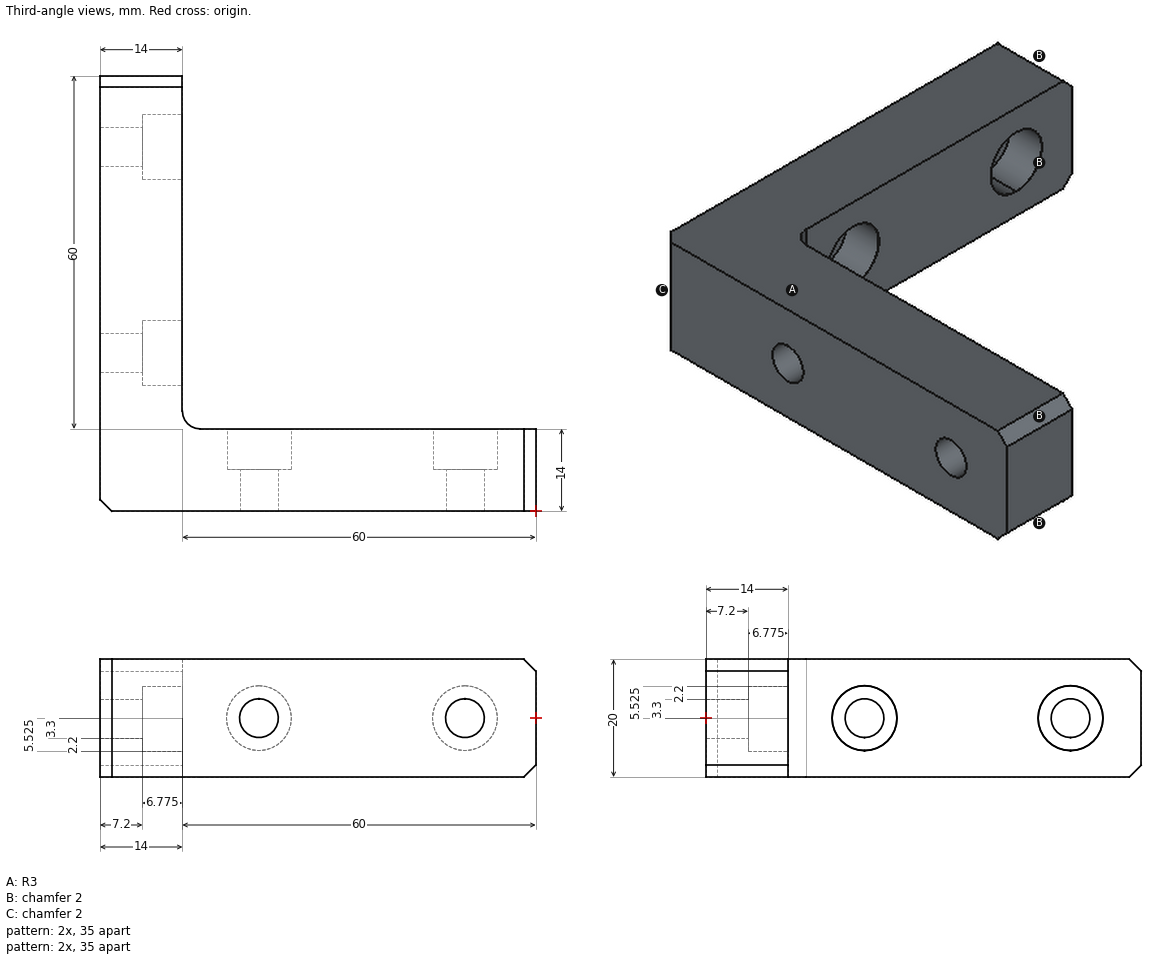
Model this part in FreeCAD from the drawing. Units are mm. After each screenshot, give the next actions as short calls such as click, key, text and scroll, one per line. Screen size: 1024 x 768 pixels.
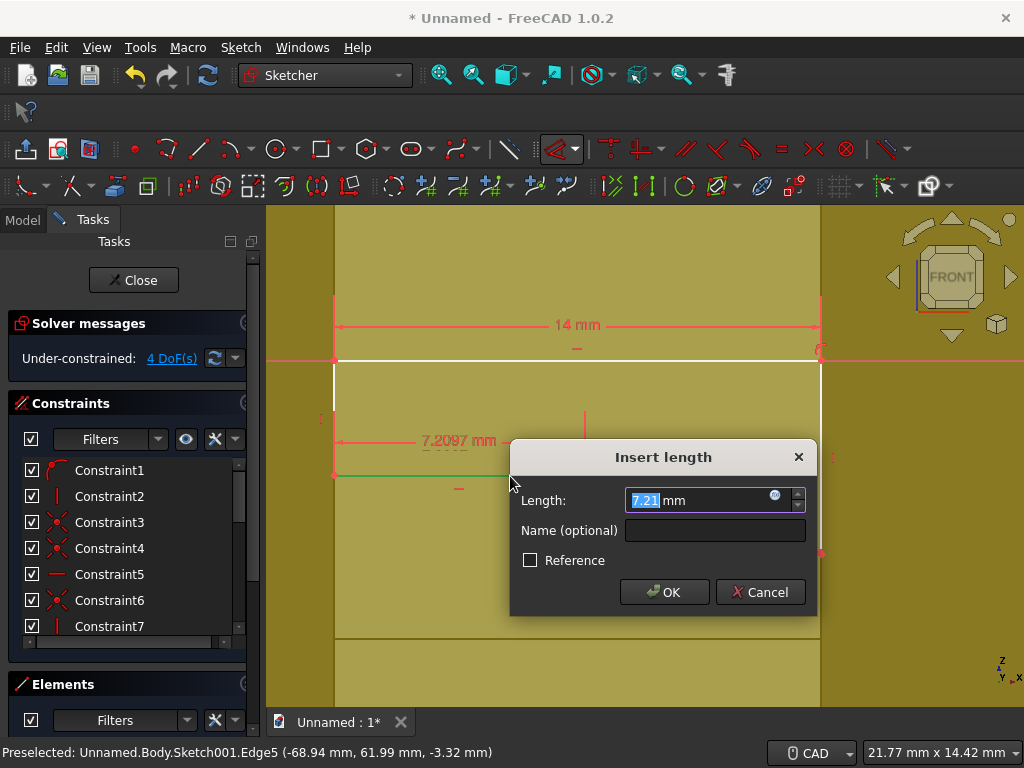
text(7.2)
key(Return)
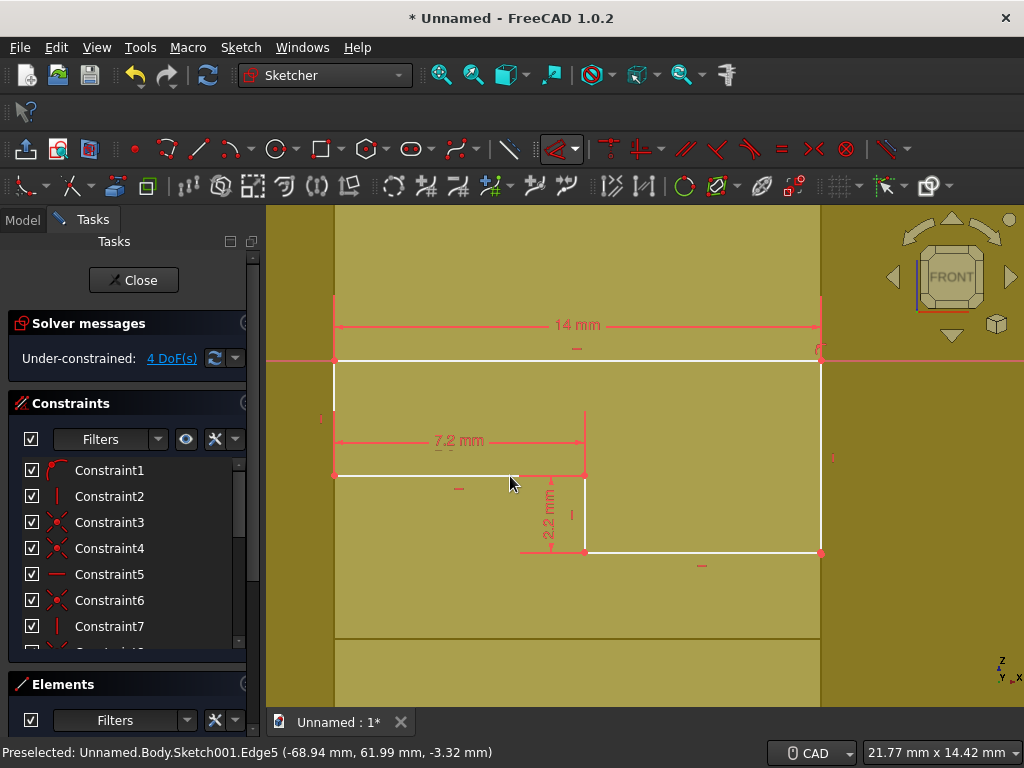
click(334, 441)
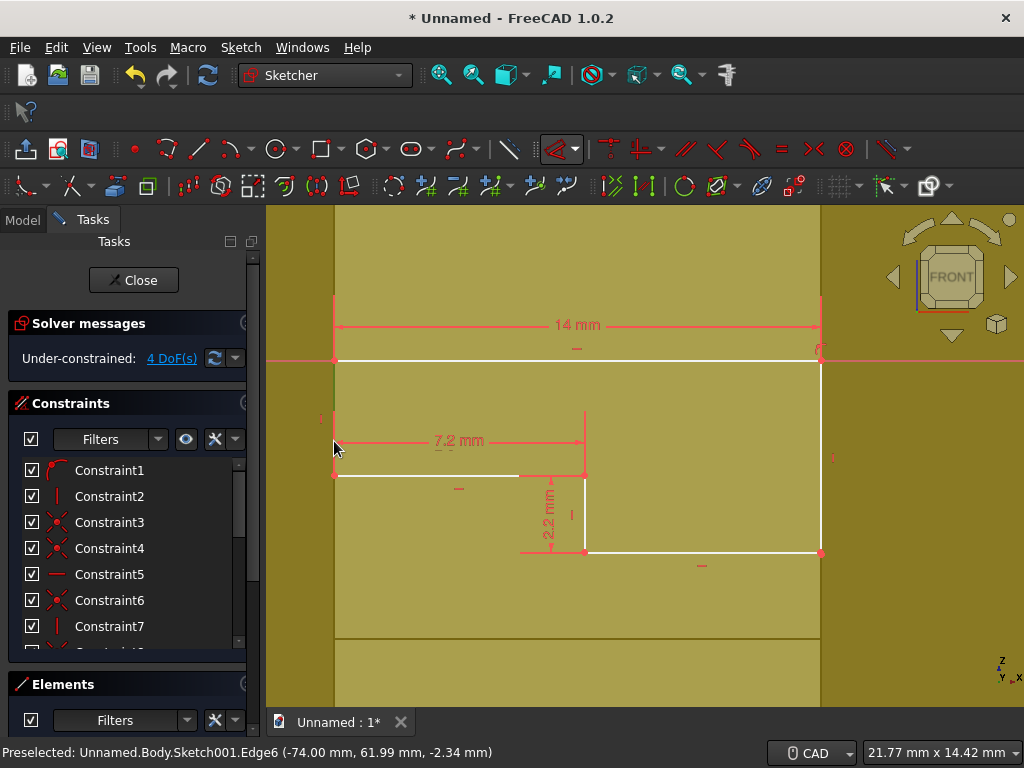
key(i)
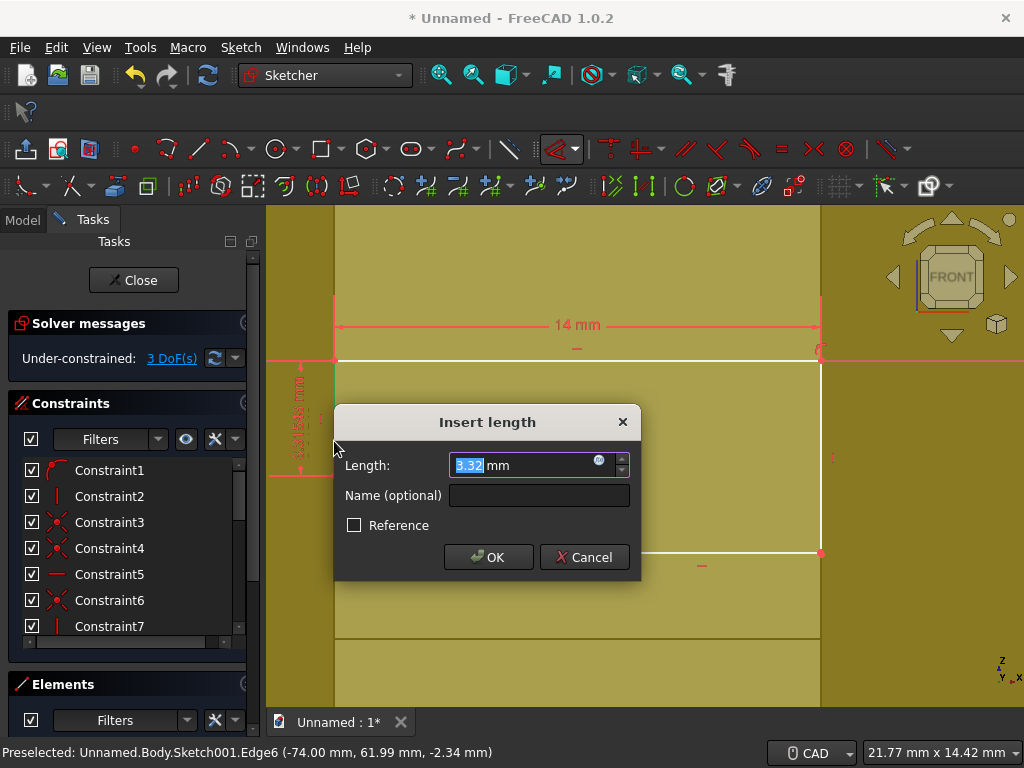
text(3.3)
key(Return)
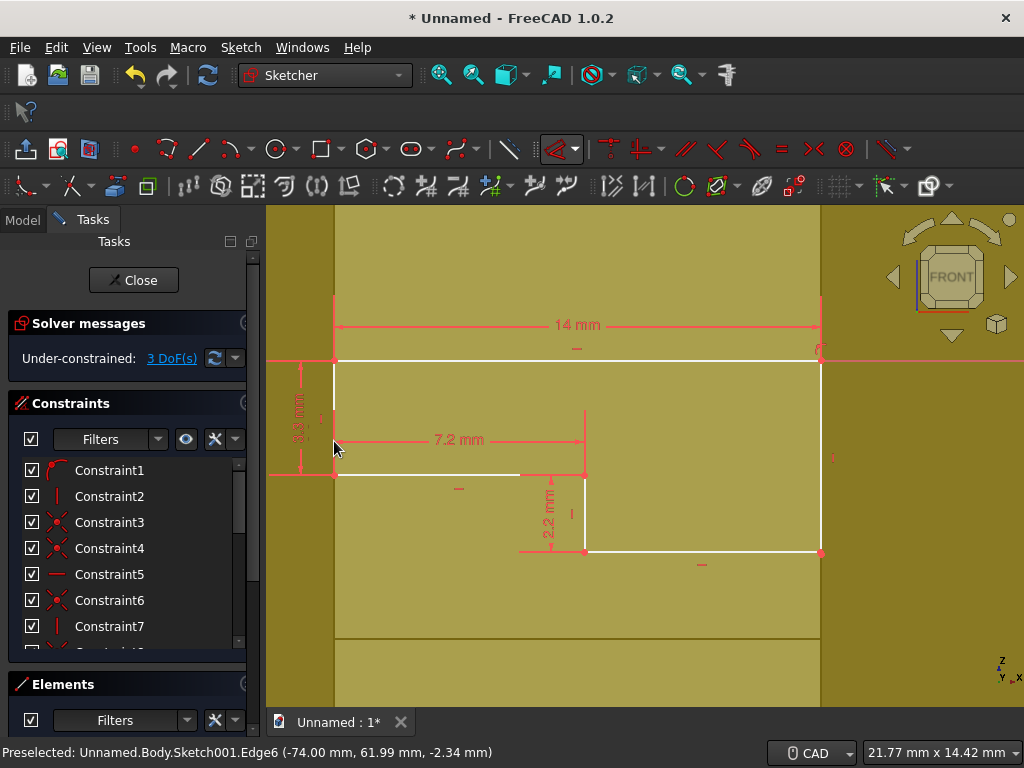
click(821, 361)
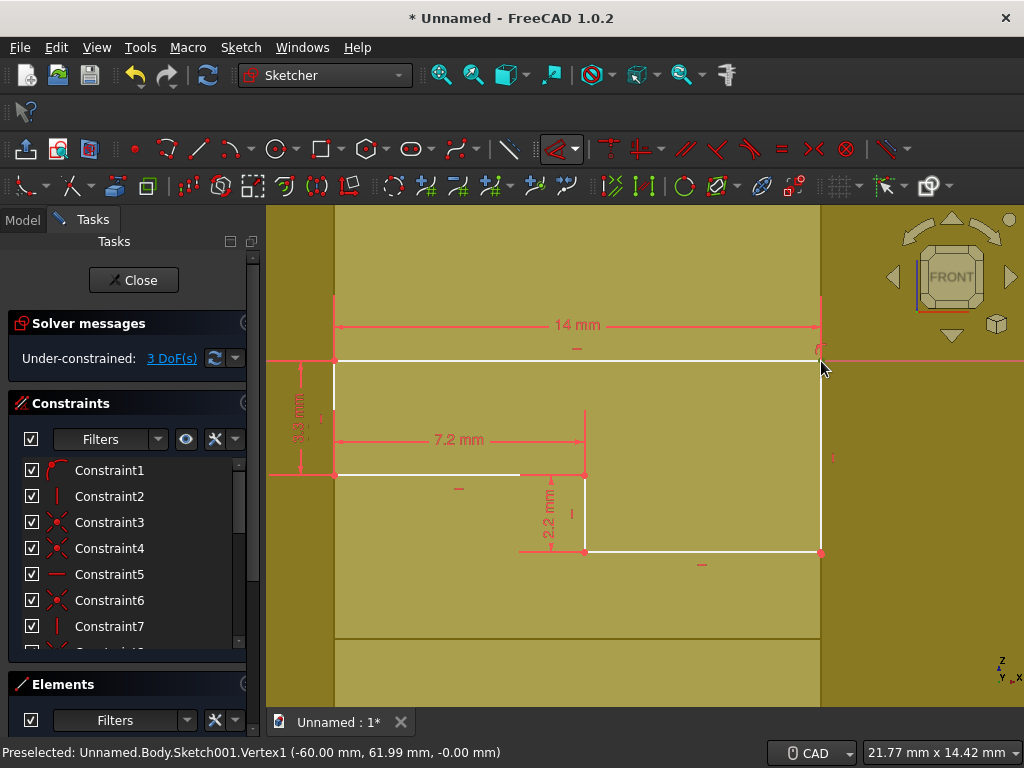
click(578, 150)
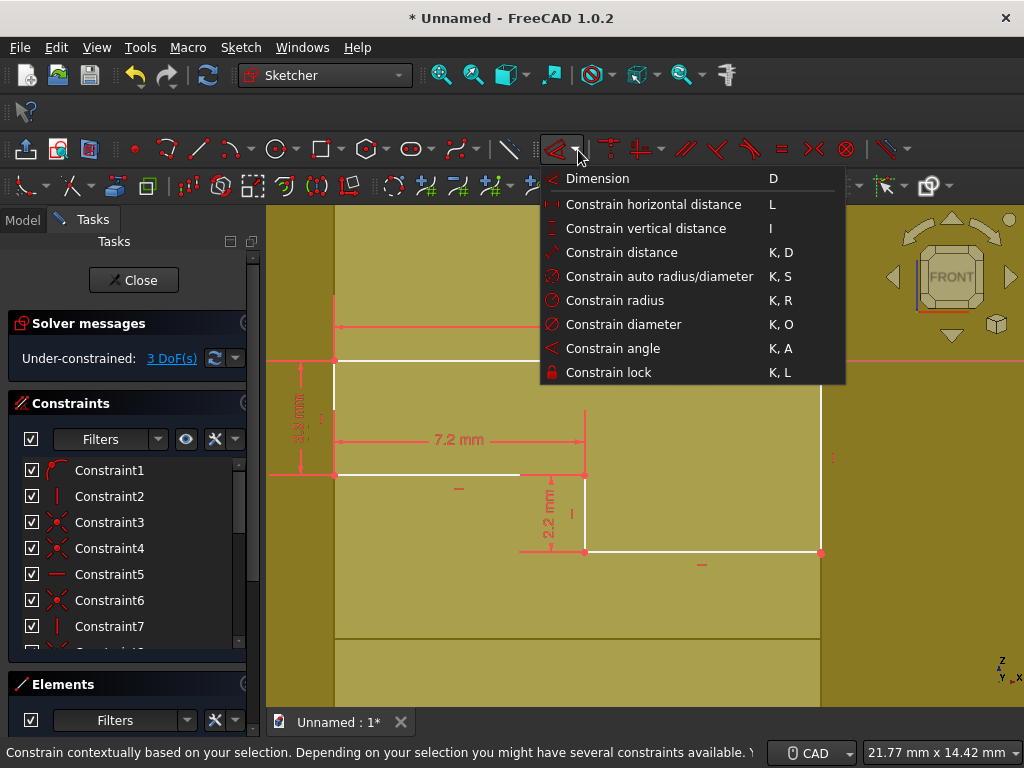
click(693, 204)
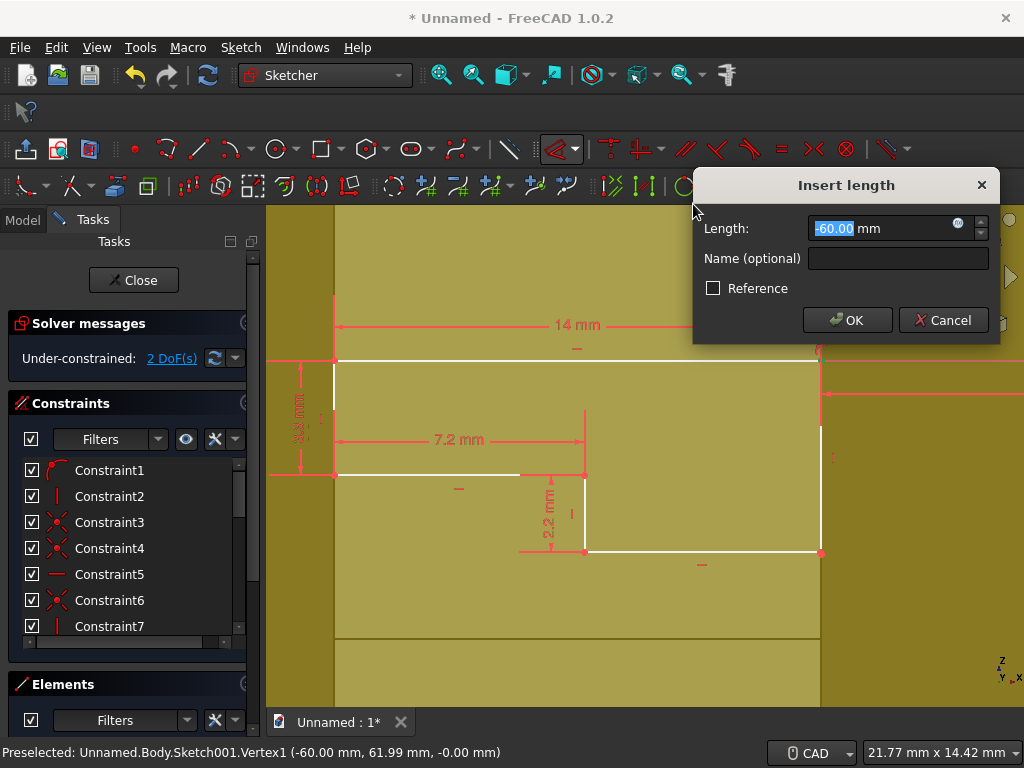
text(-60)
key(Return)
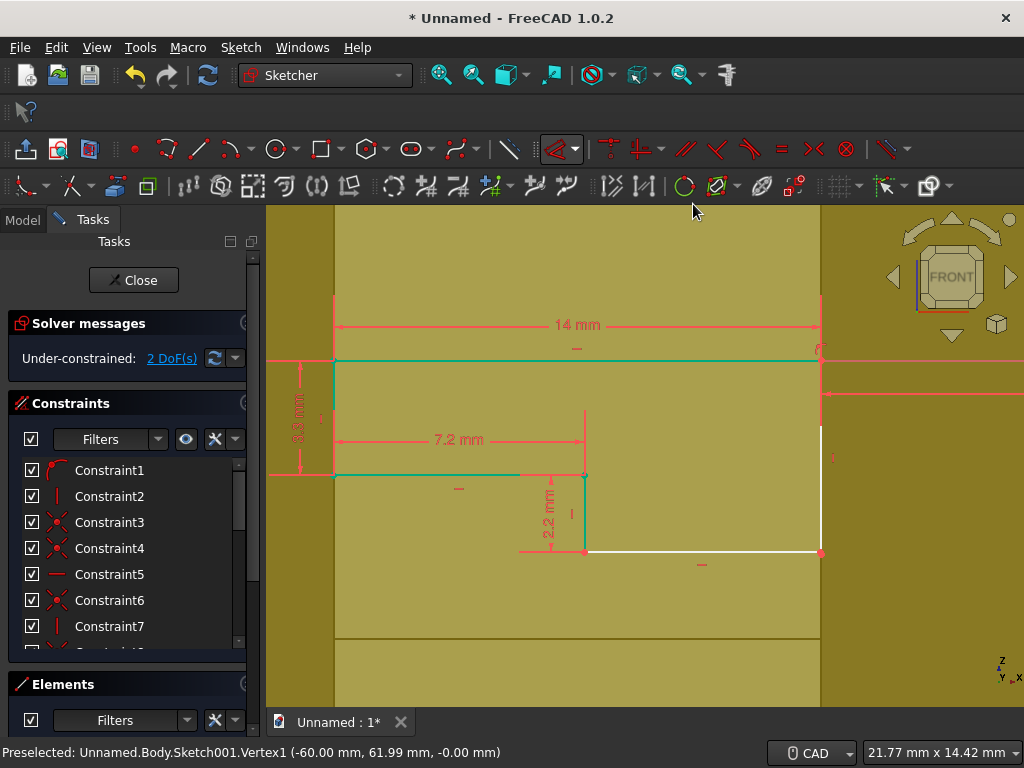
click(821, 419)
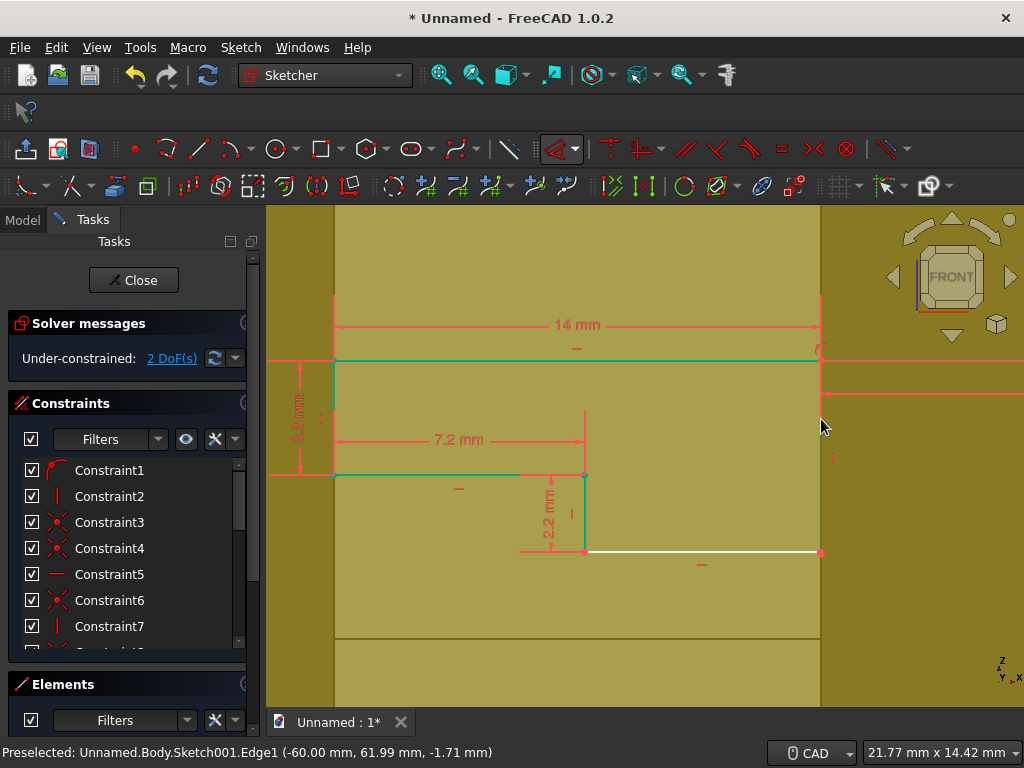
click(578, 150)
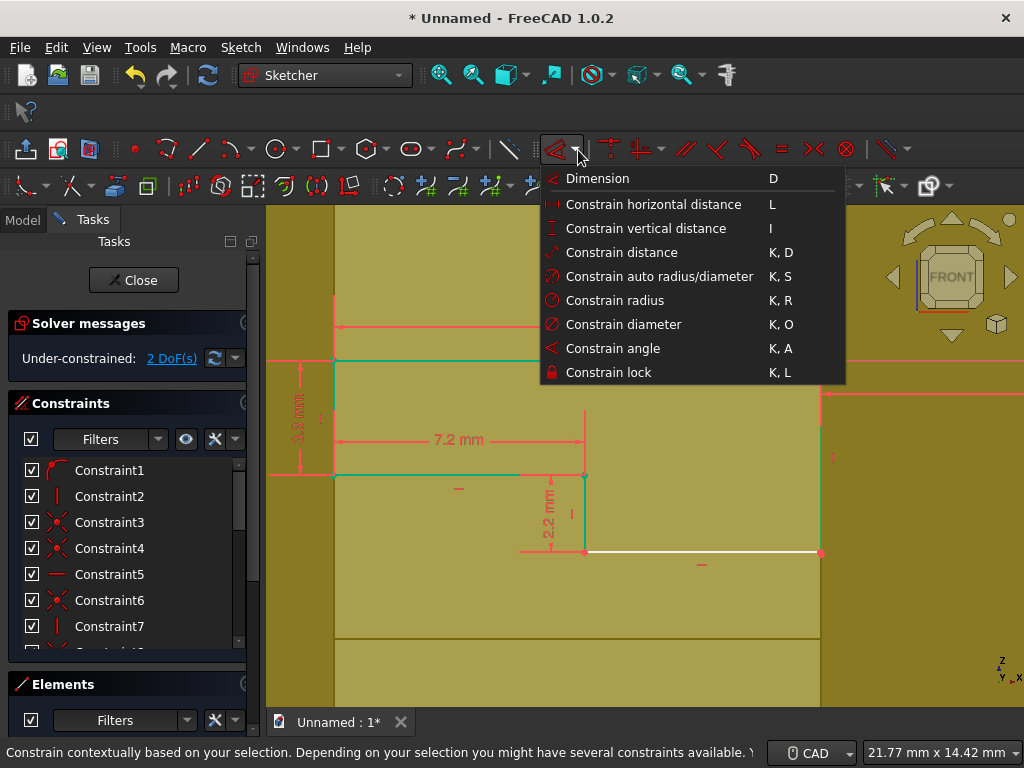
click(693, 228)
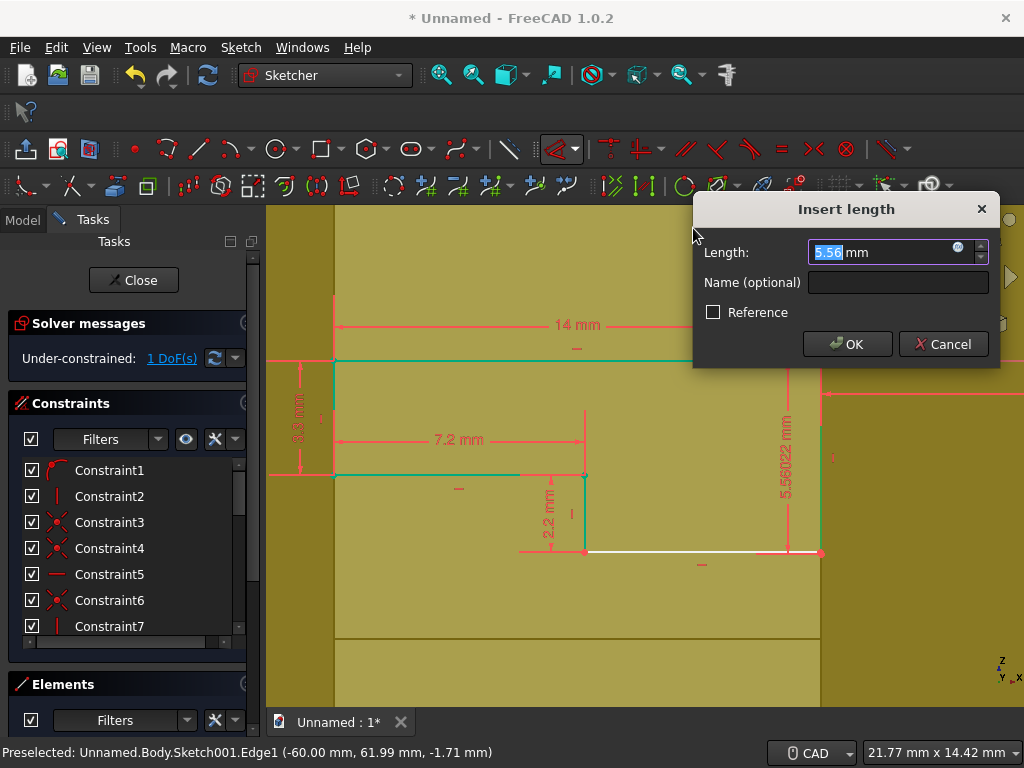
text(5.525)
key(Return)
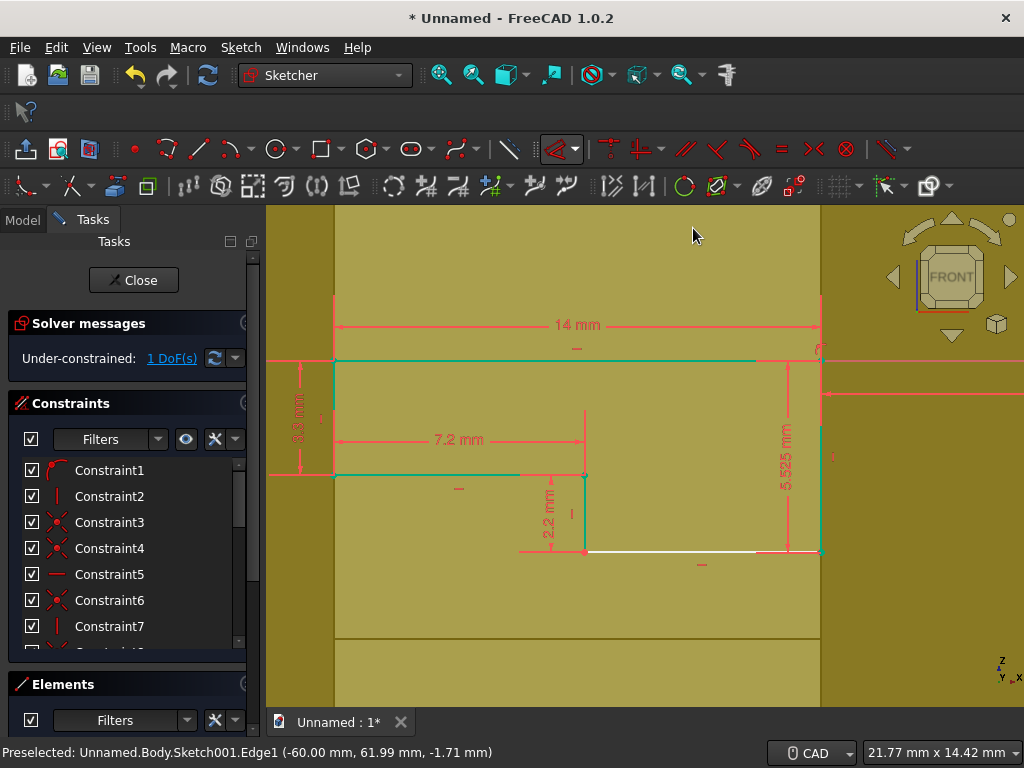
click(750, 552)